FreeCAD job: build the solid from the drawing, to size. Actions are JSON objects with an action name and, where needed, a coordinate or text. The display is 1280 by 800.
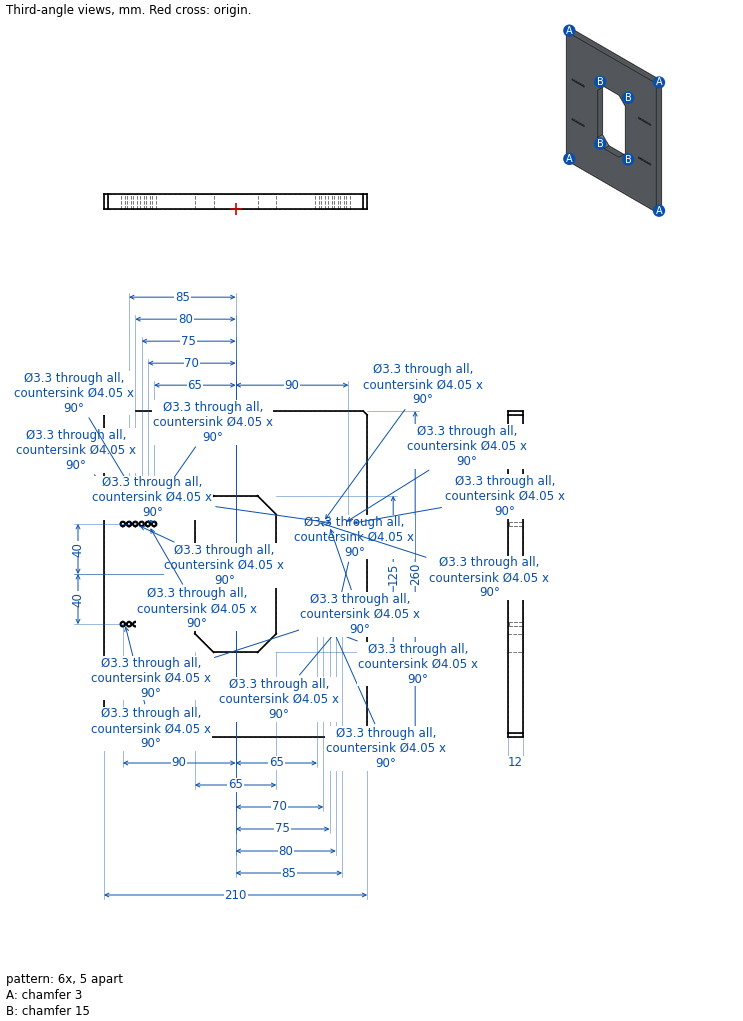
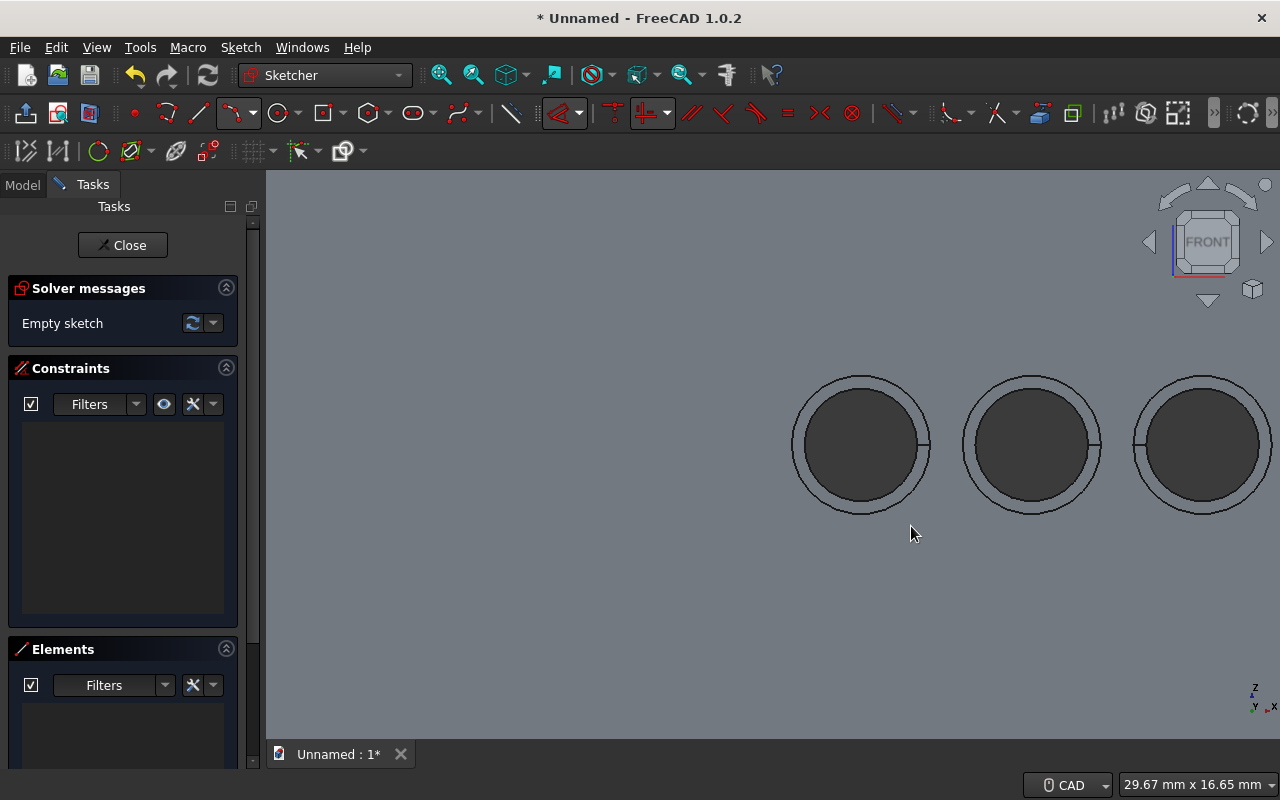
{"action": "scroll", "coordinate": [684, 441], "scroll_direction": "up", "scroll_amount": 6}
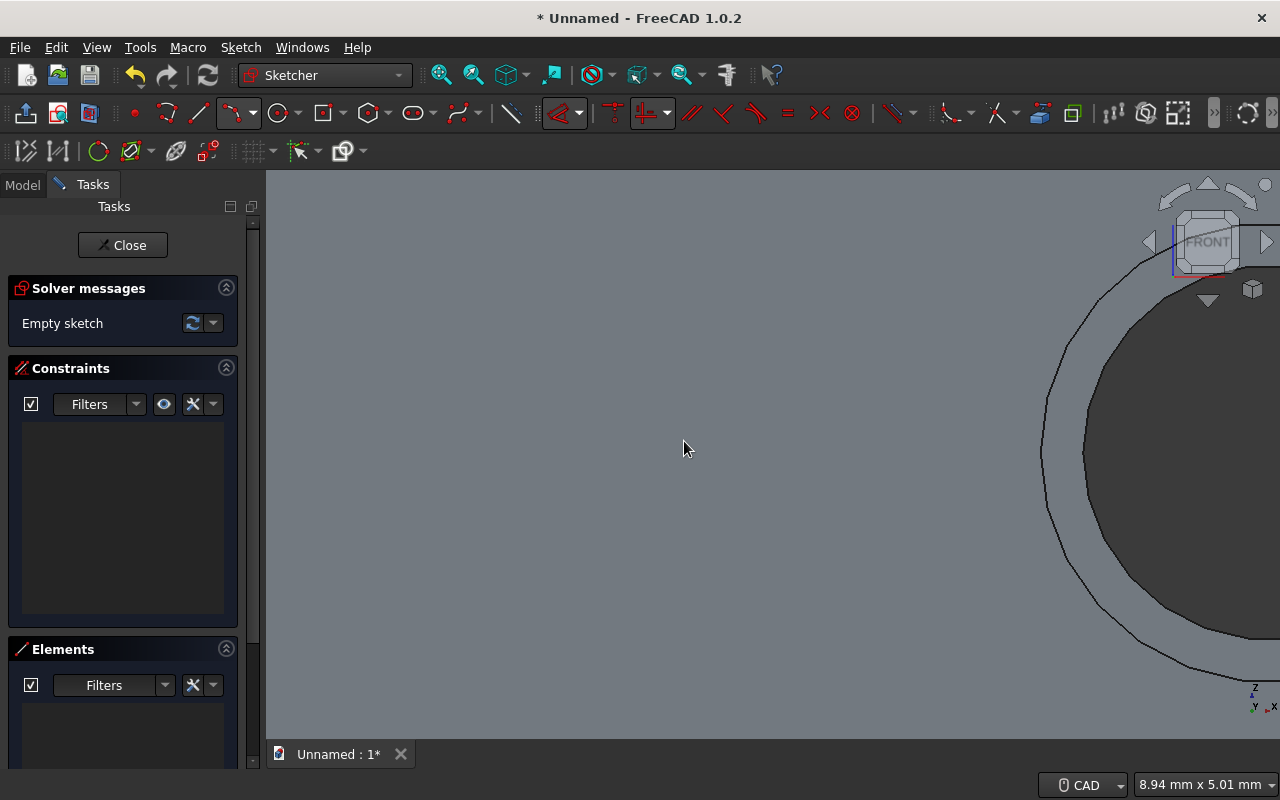
{"action": "left_click", "coordinate": [278, 114]}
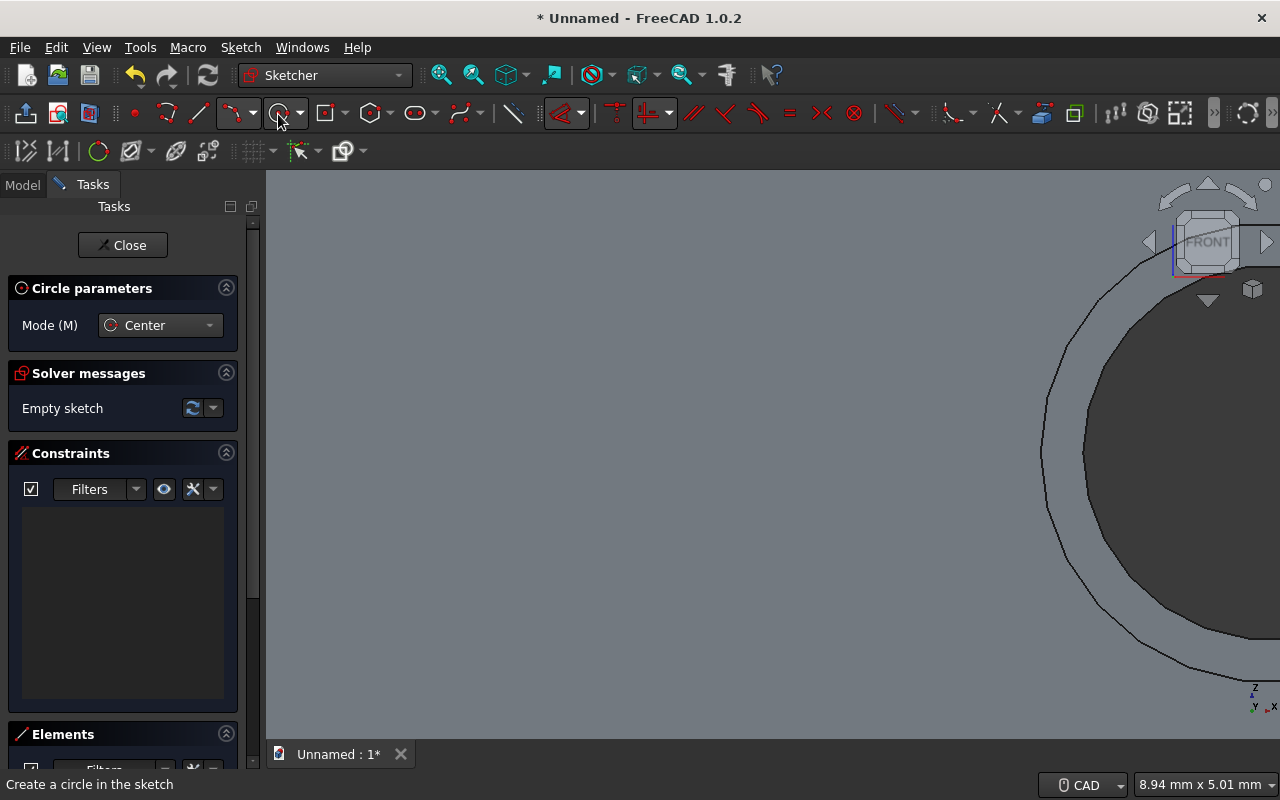
{"action": "left_click", "coordinate": [703, 453]}
{"action": "mouse_move", "coordinate": [836, 320]}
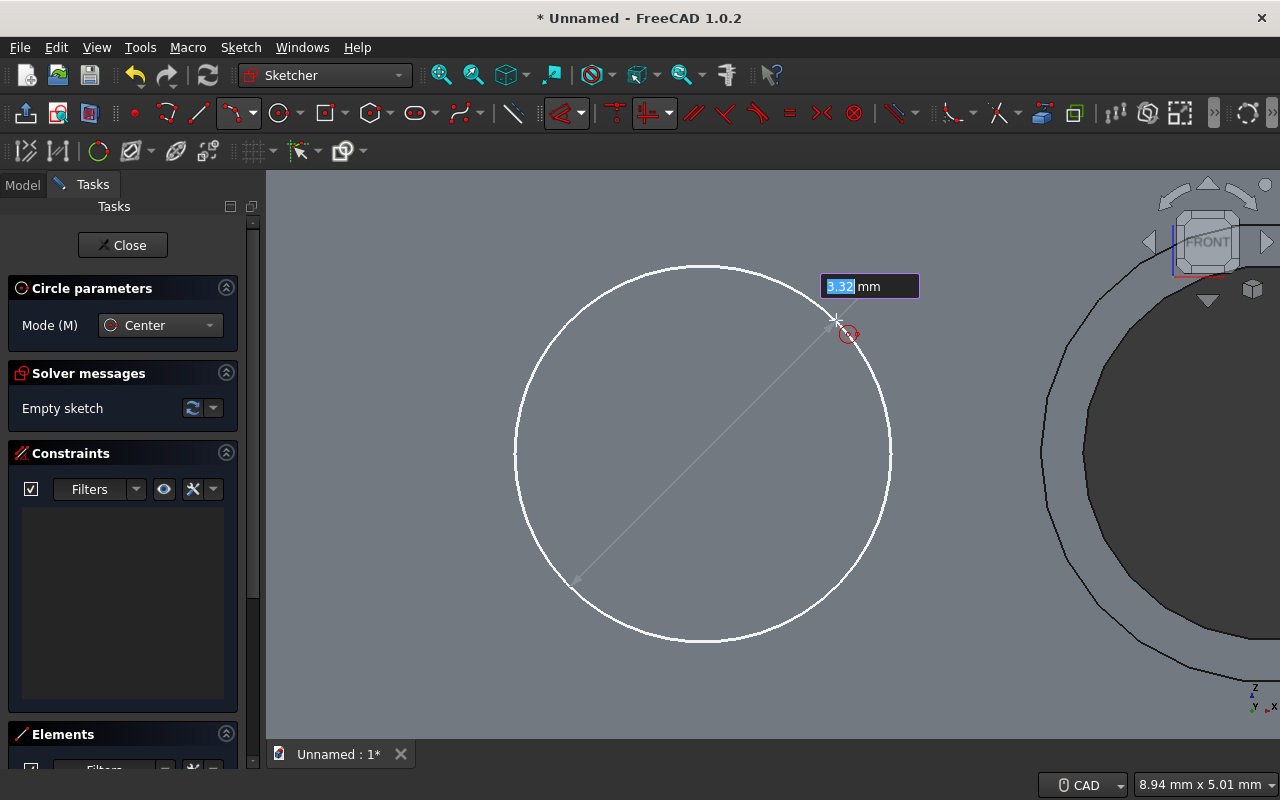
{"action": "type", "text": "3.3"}
{"action": "key", "text": "Return"}
{"action": "key", "text": "Escape"}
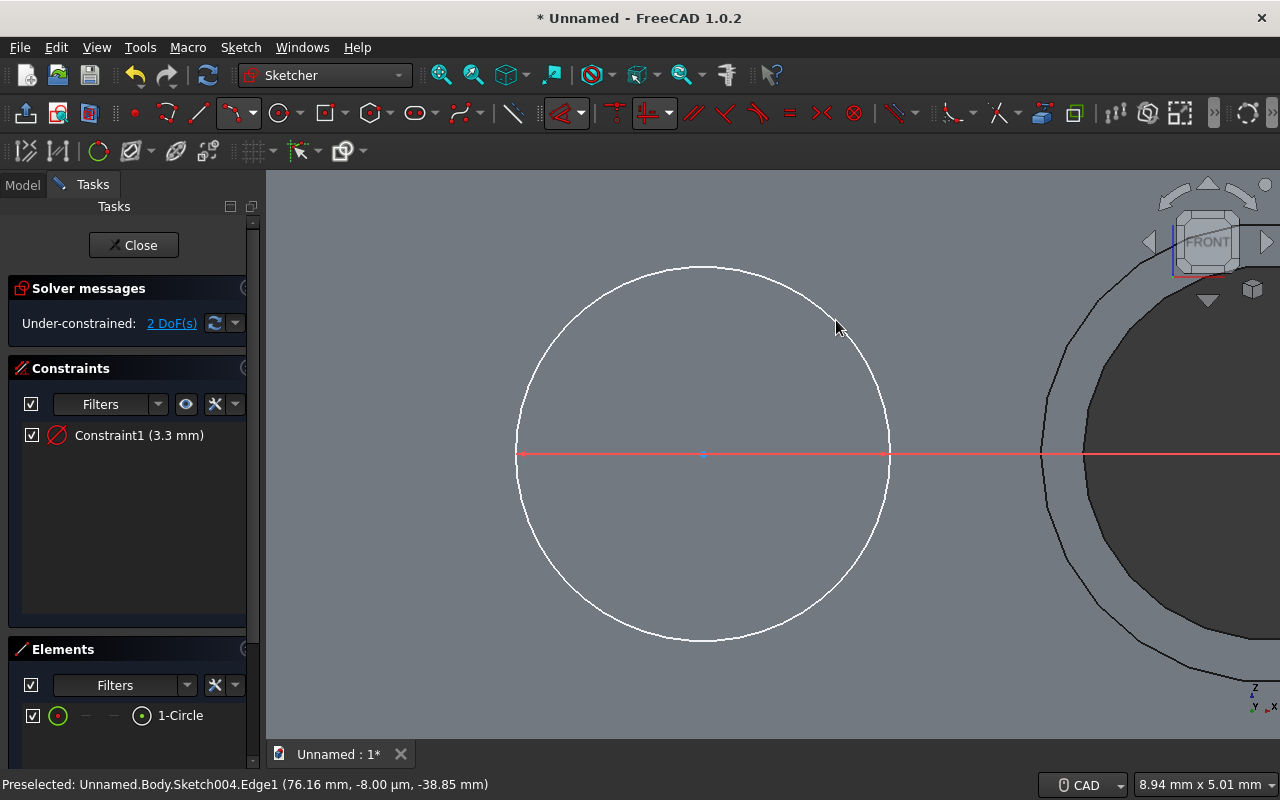
{"action": "left_click", "coordinate": [703, 454]}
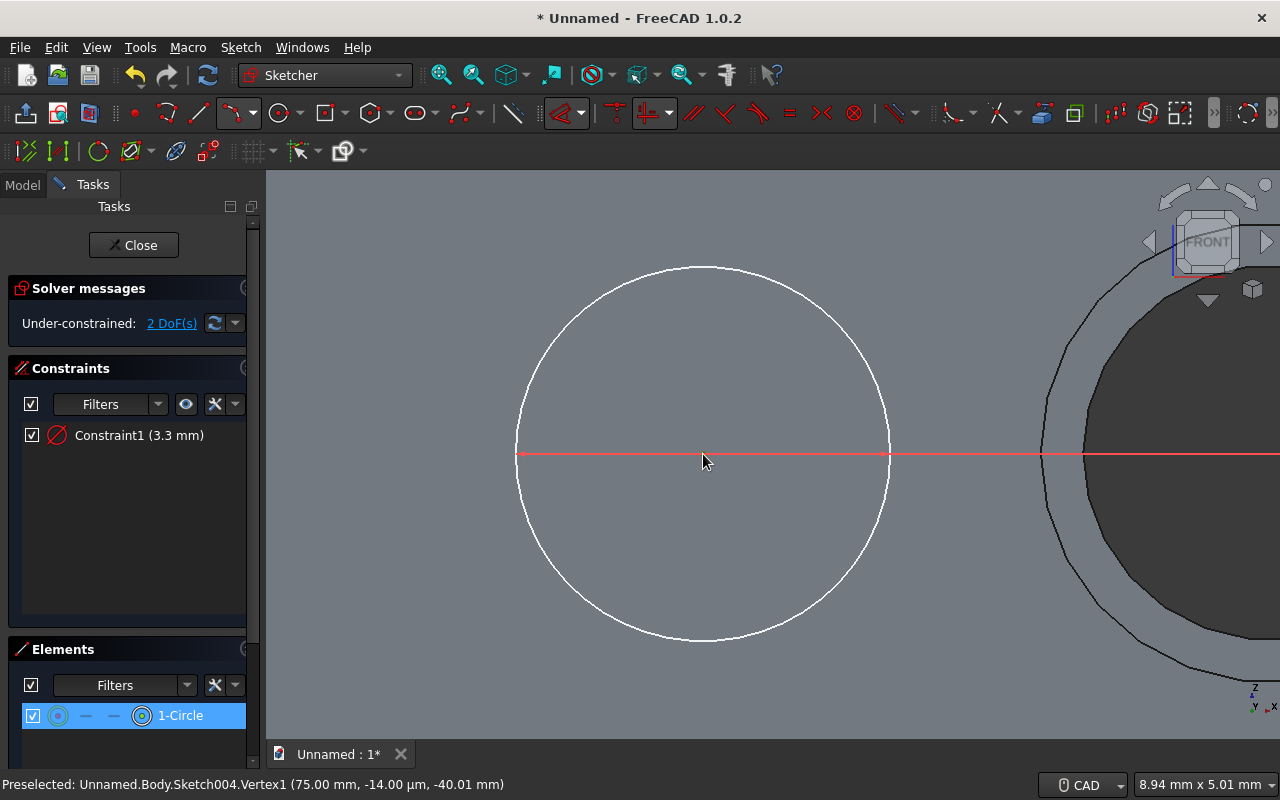
{"action": "left_click", "coordinate": [584, 114]}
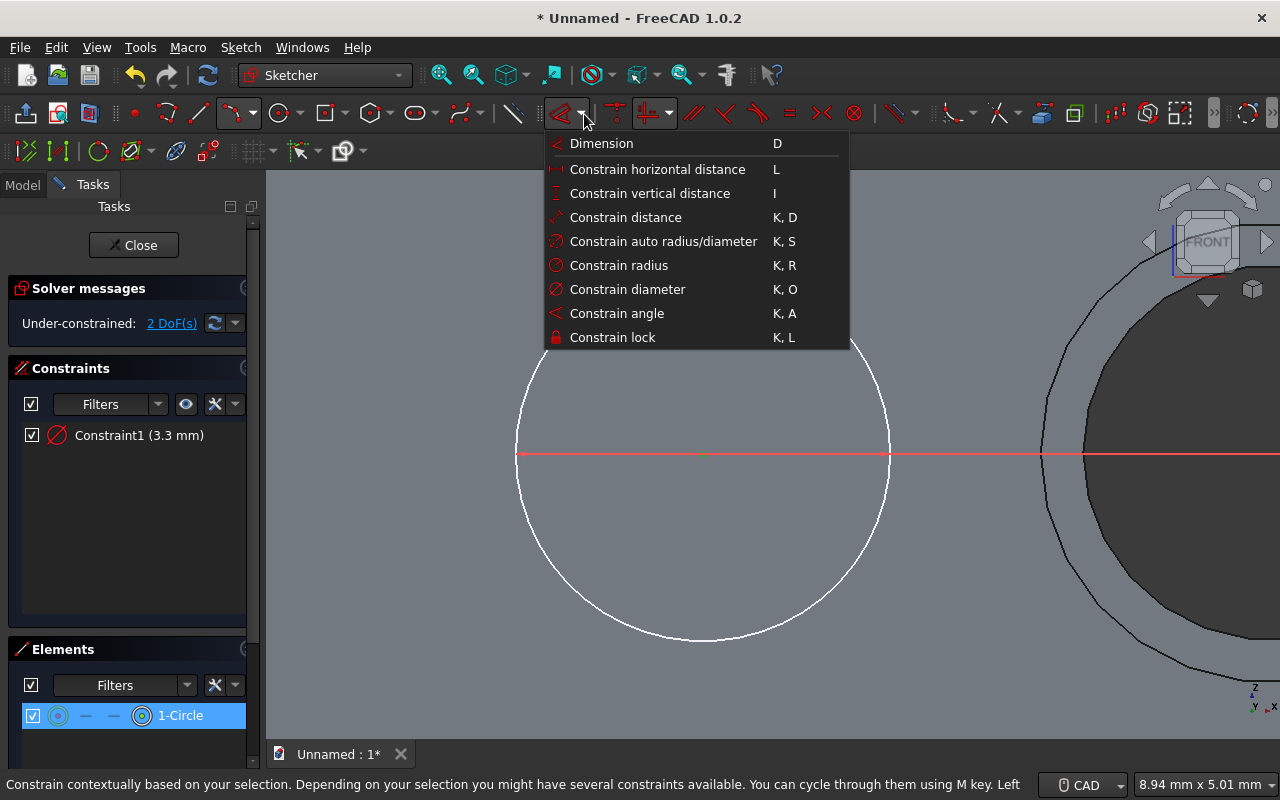
{"action": "left_click", "coordinate": [697, 169]}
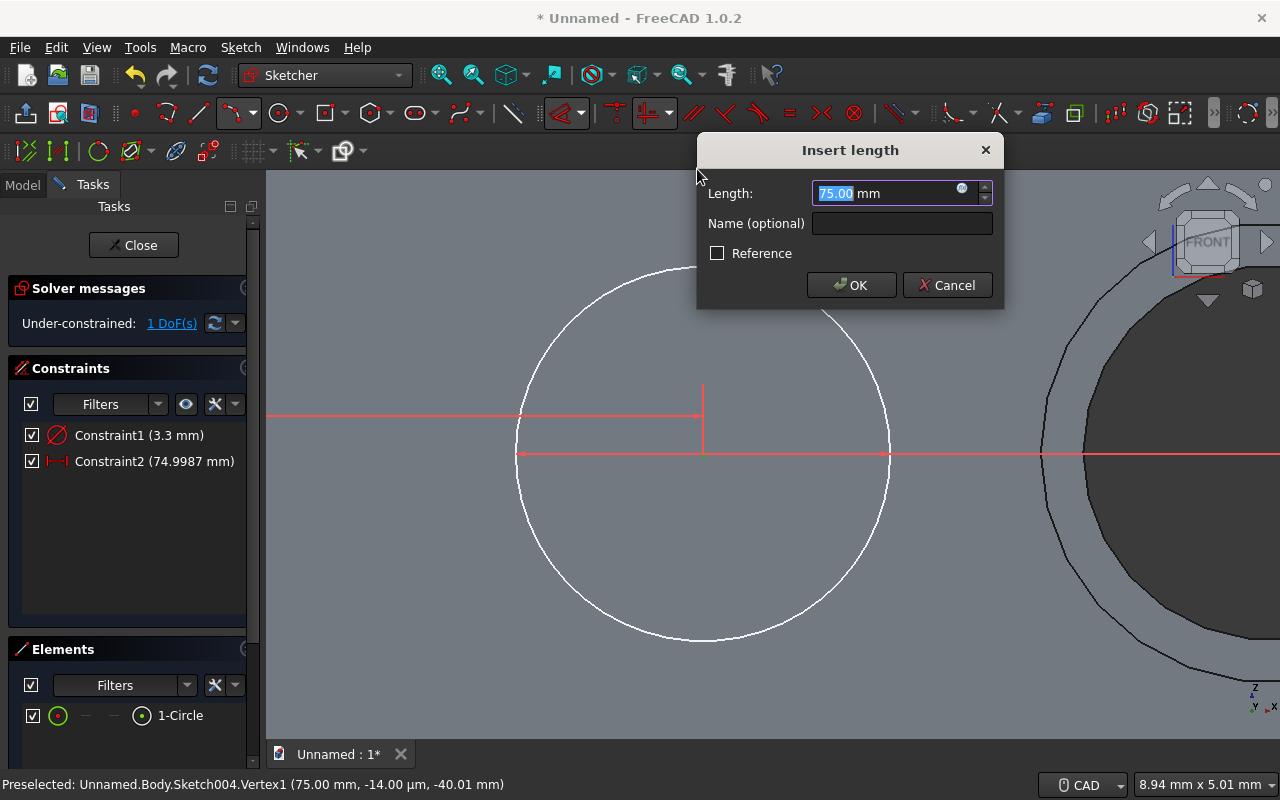
{"action": "type", "text": "75"}
{"action": "key", "text": "Return"}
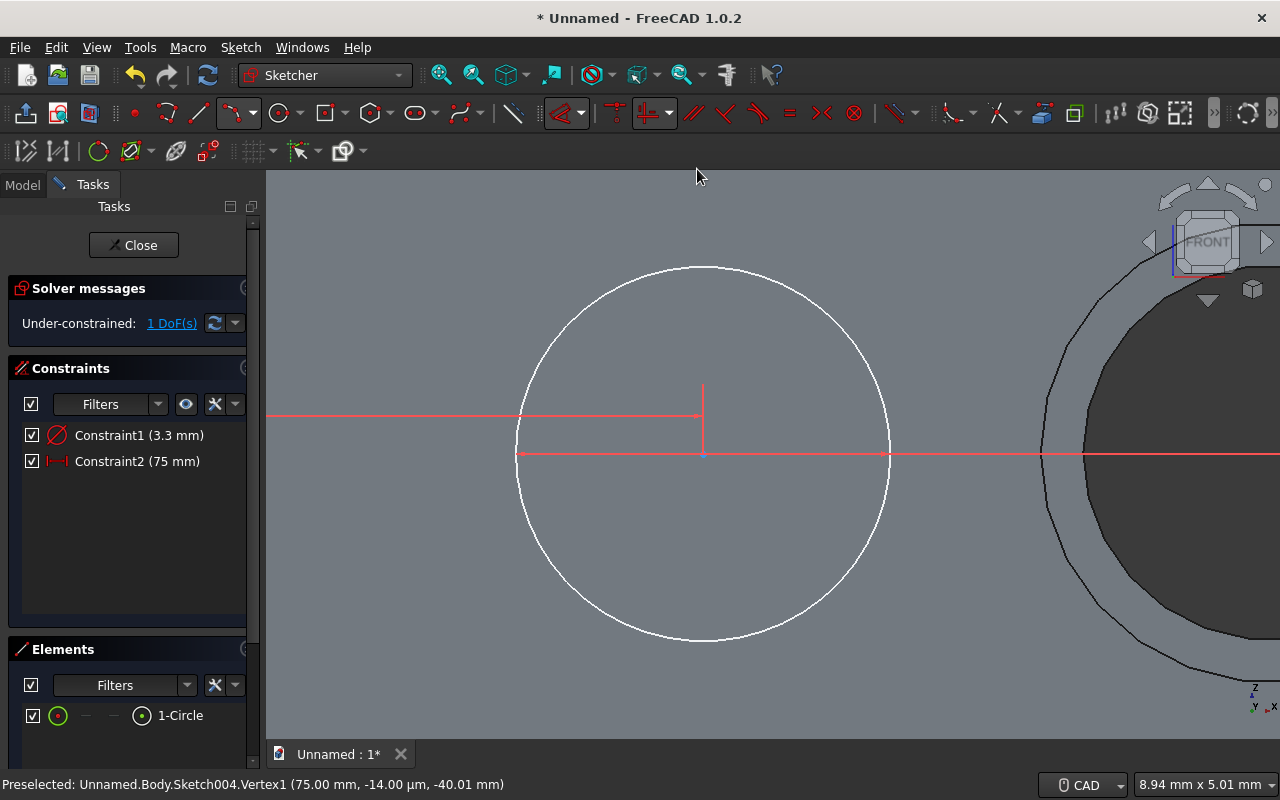
{"action": "left_click", "coordinate": [703, 454]}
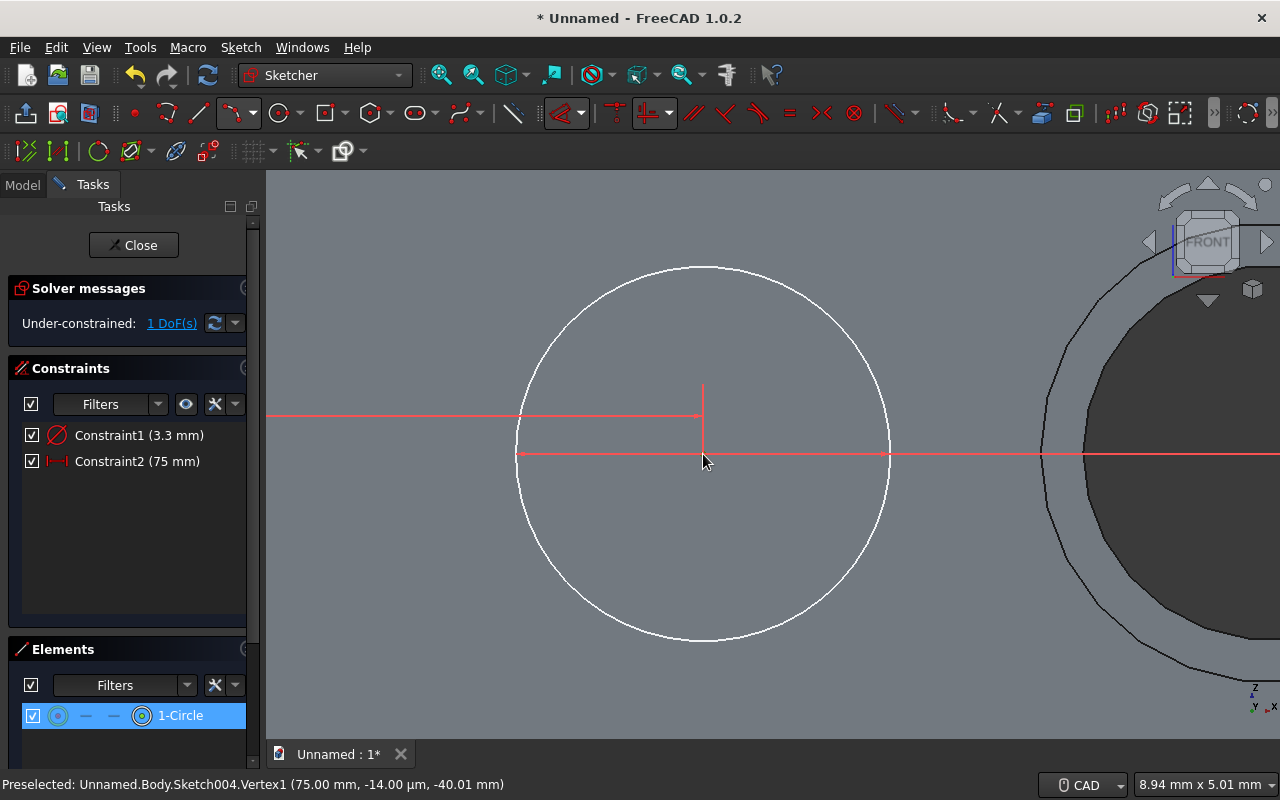
{"action": "key", "text": "i"}